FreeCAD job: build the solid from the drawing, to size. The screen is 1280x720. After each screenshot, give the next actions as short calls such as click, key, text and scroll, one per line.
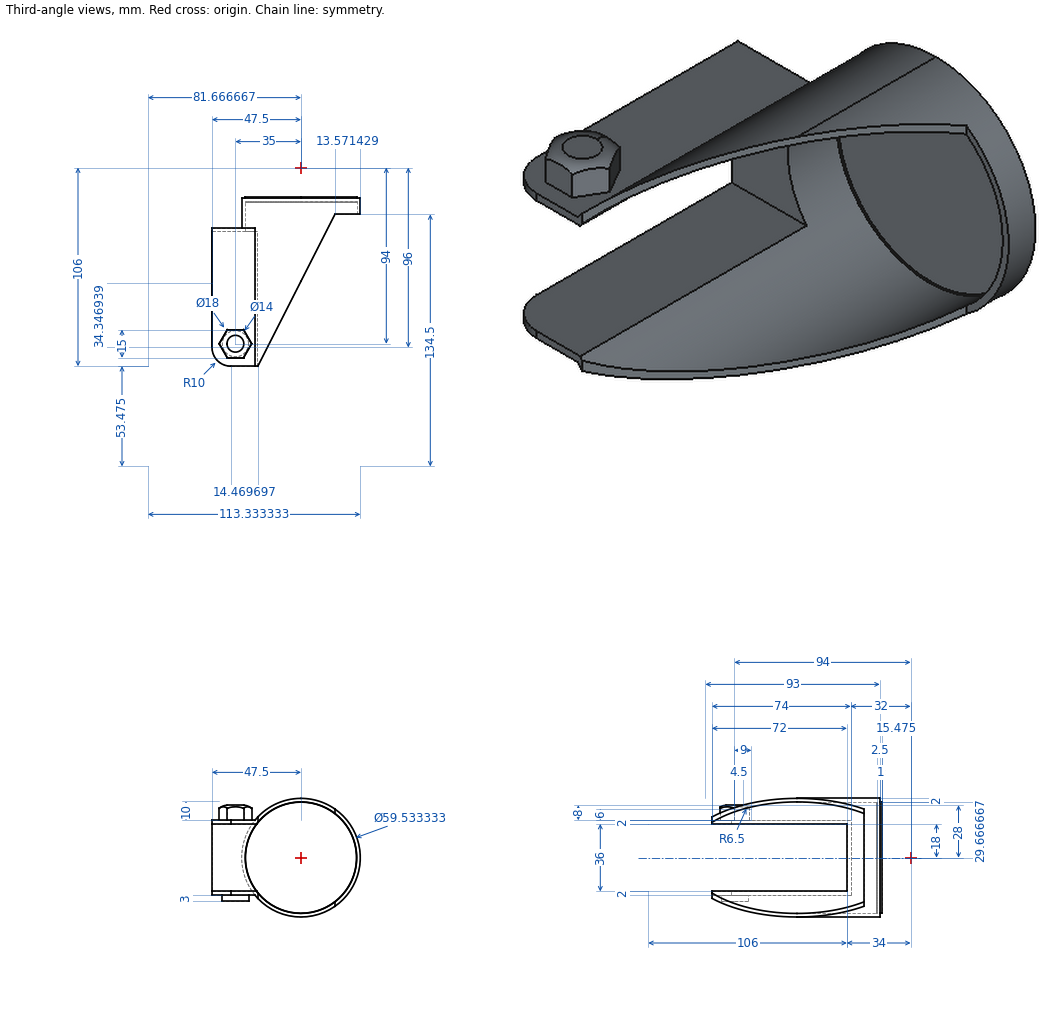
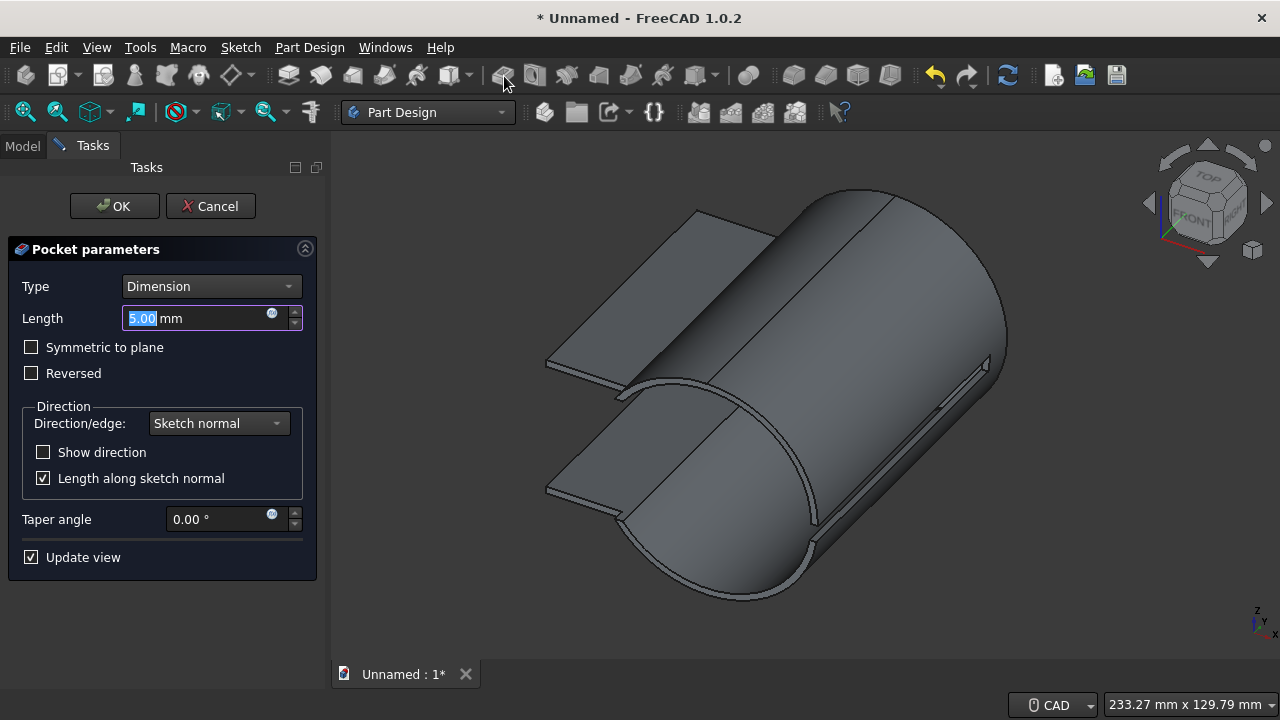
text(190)
key(Tab)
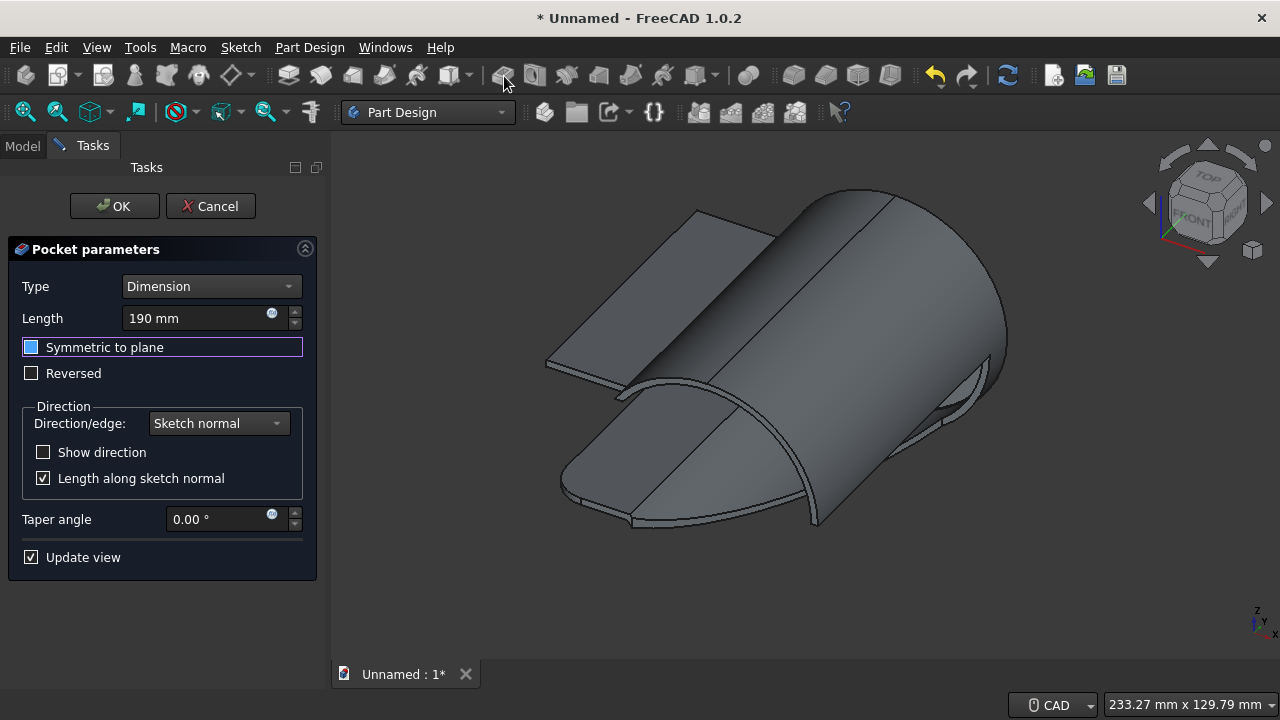
click(30, 347)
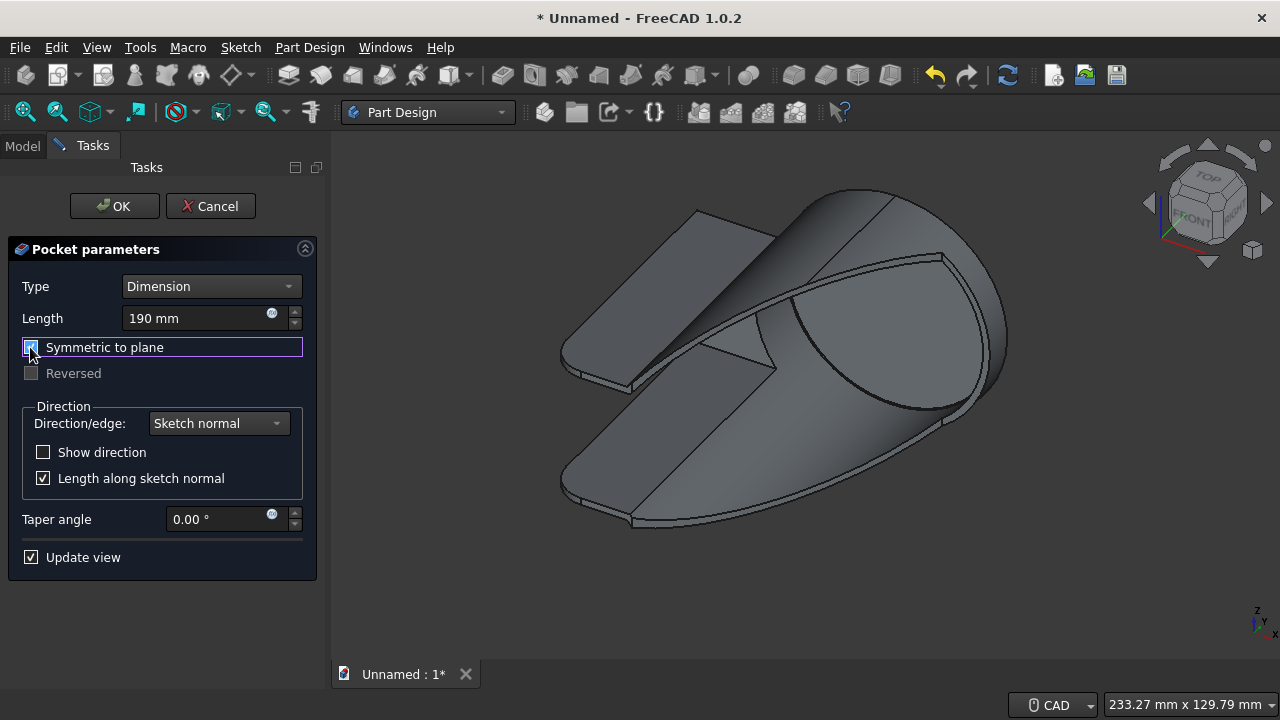
click(115, 206)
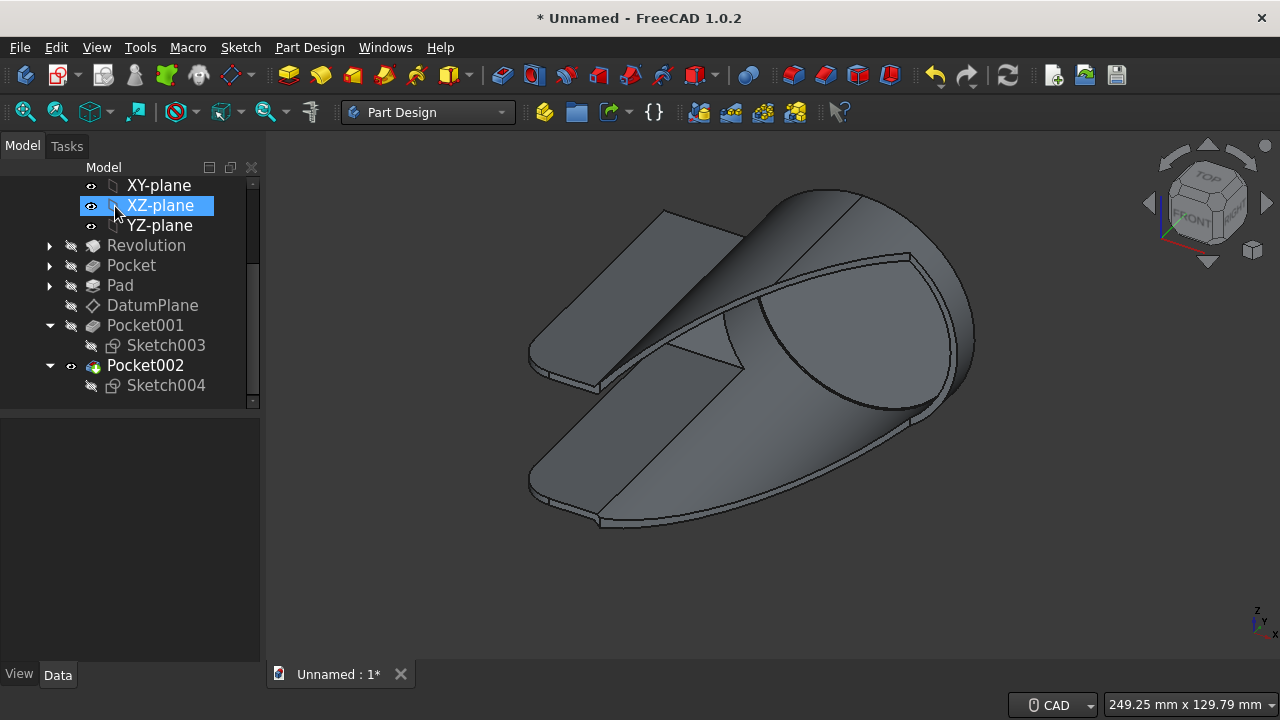
key(5)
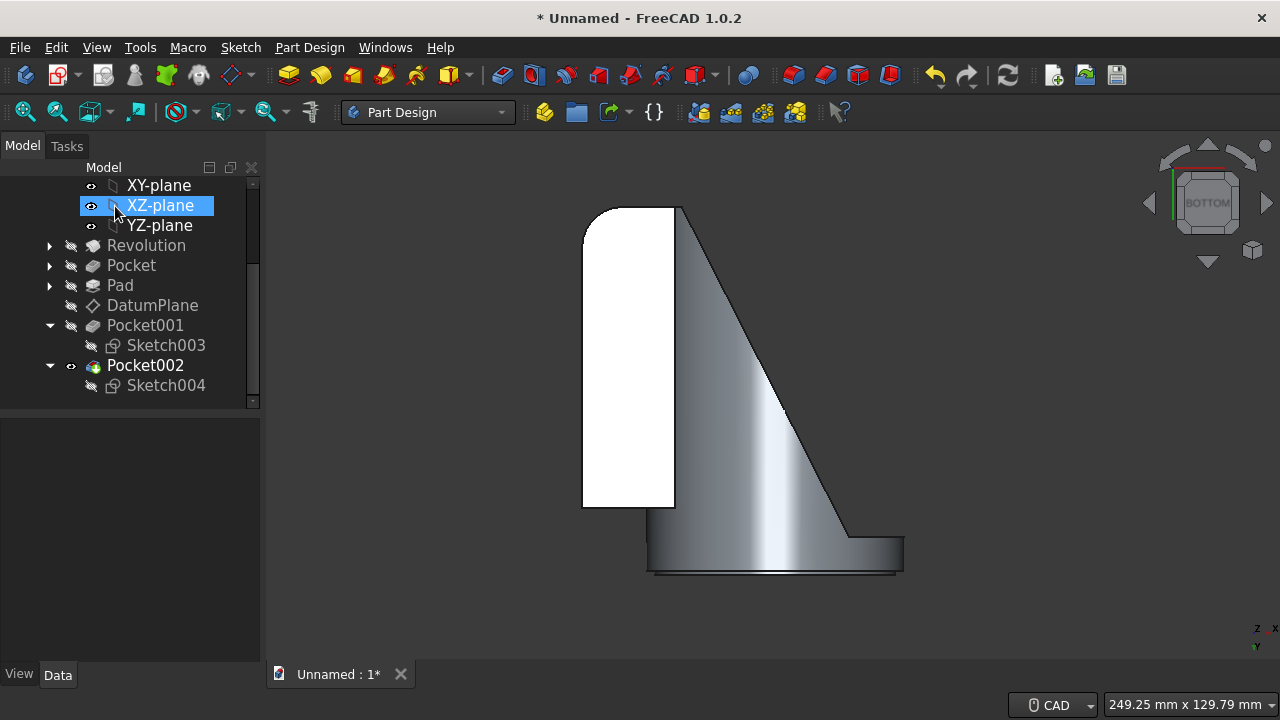
click(629, 443)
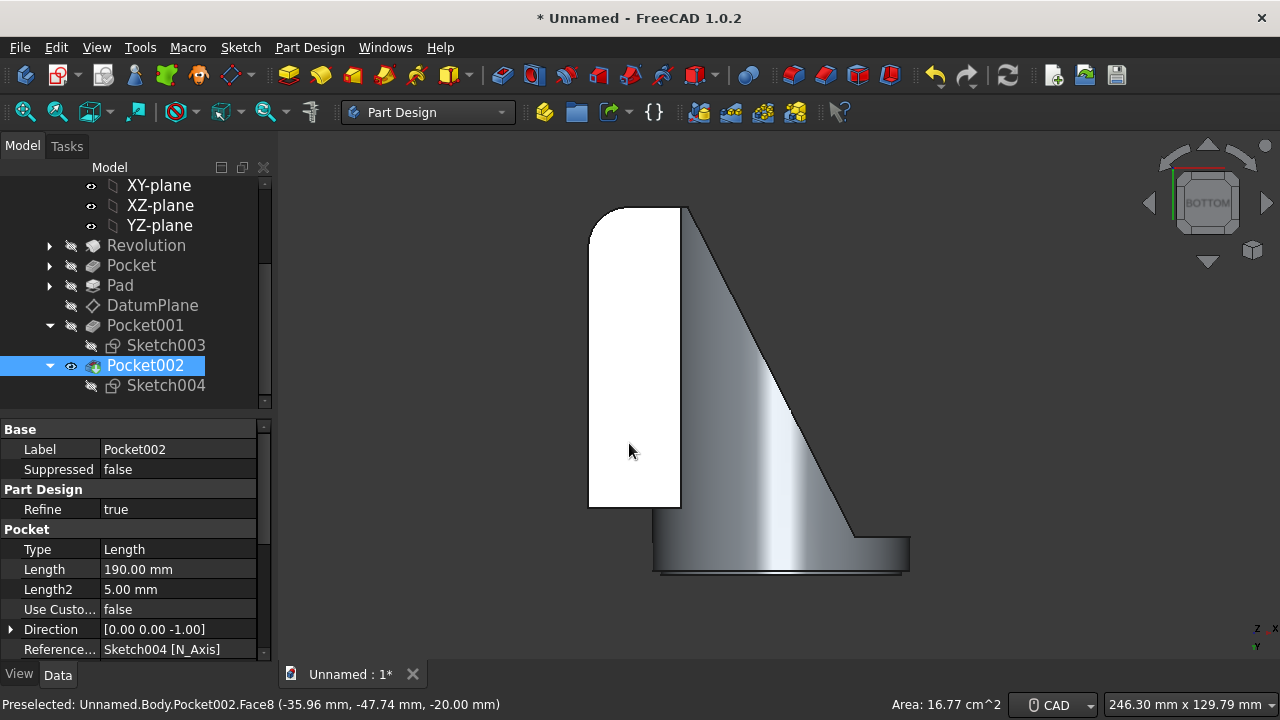
click(58, 76)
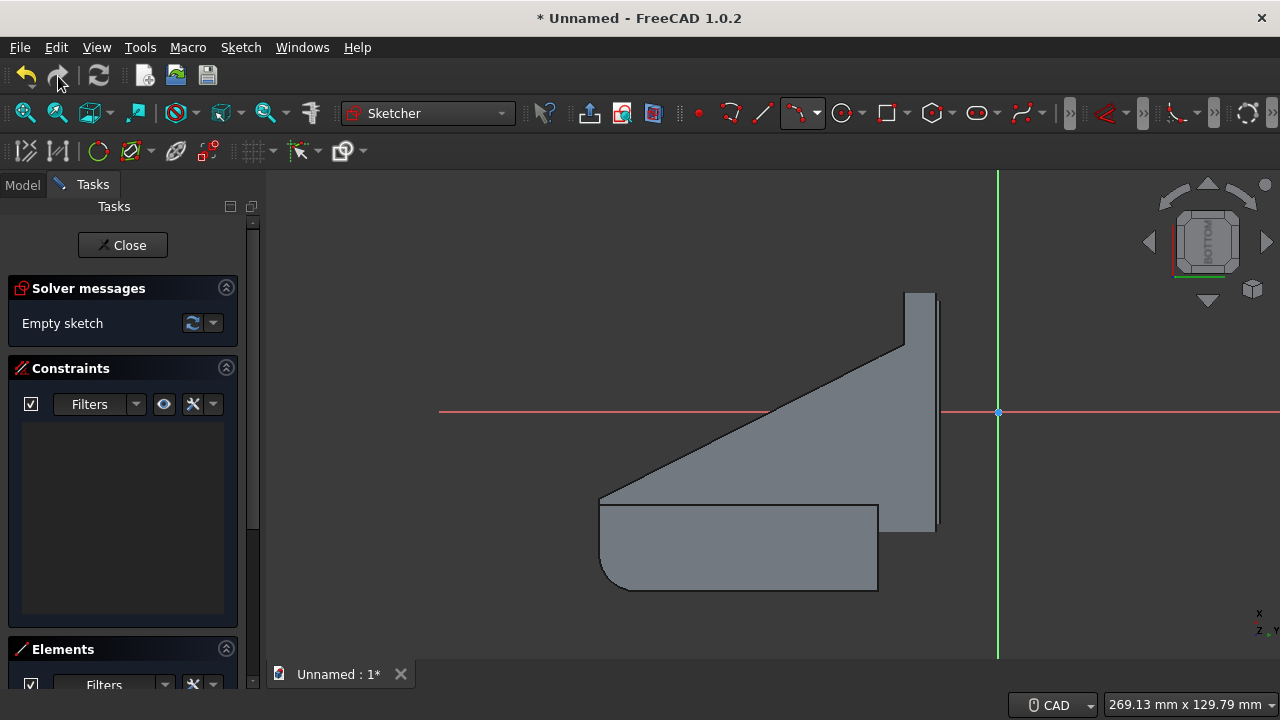
key(q)
key(s)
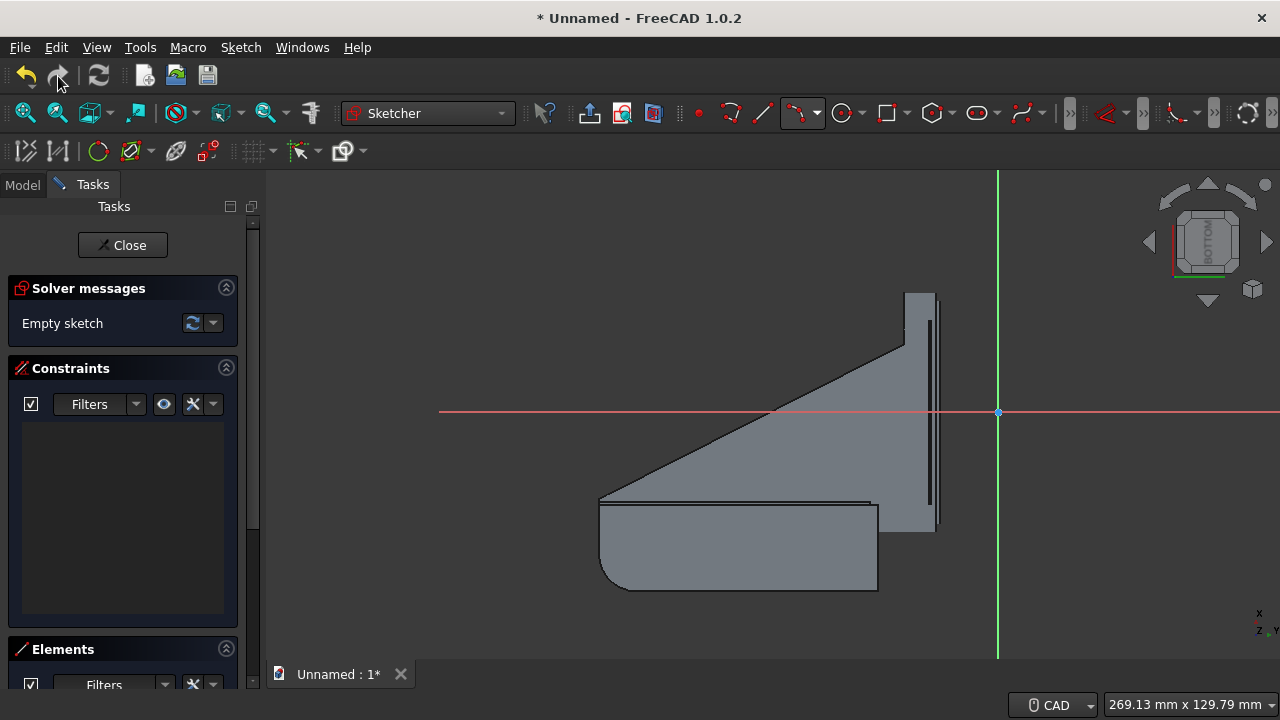
scroll(632, 570, up, 9)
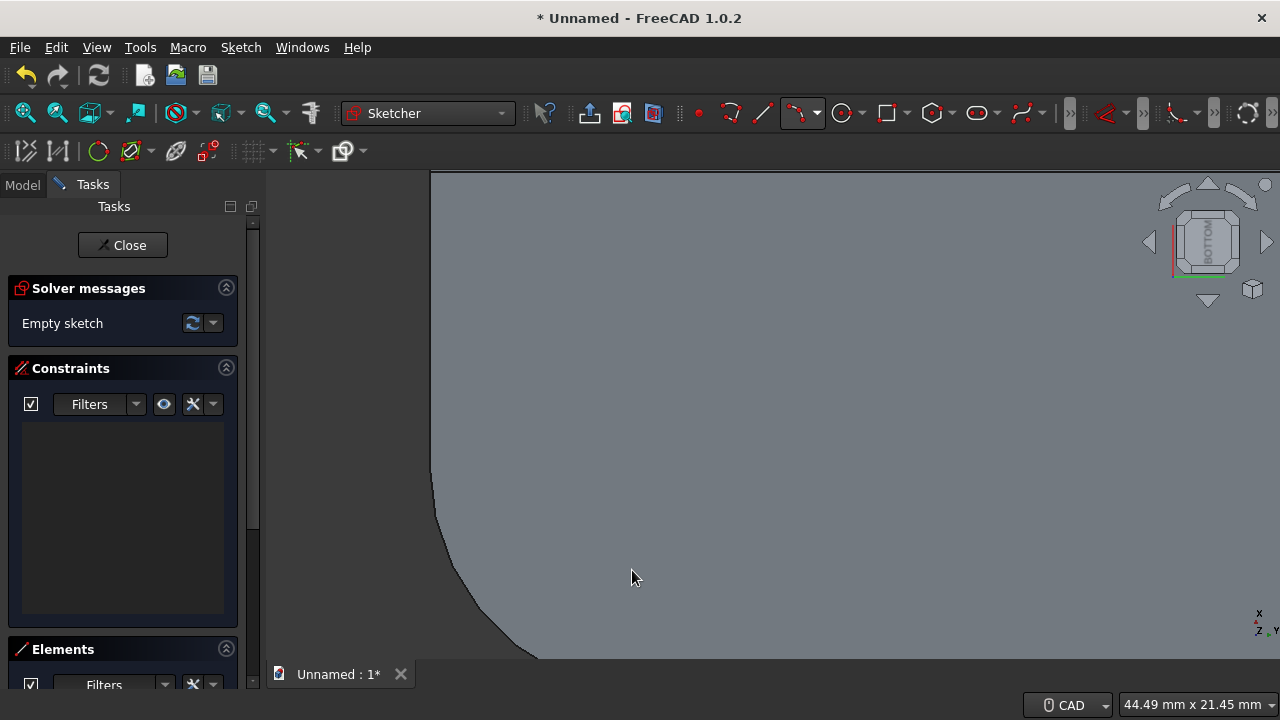
click(842, 114)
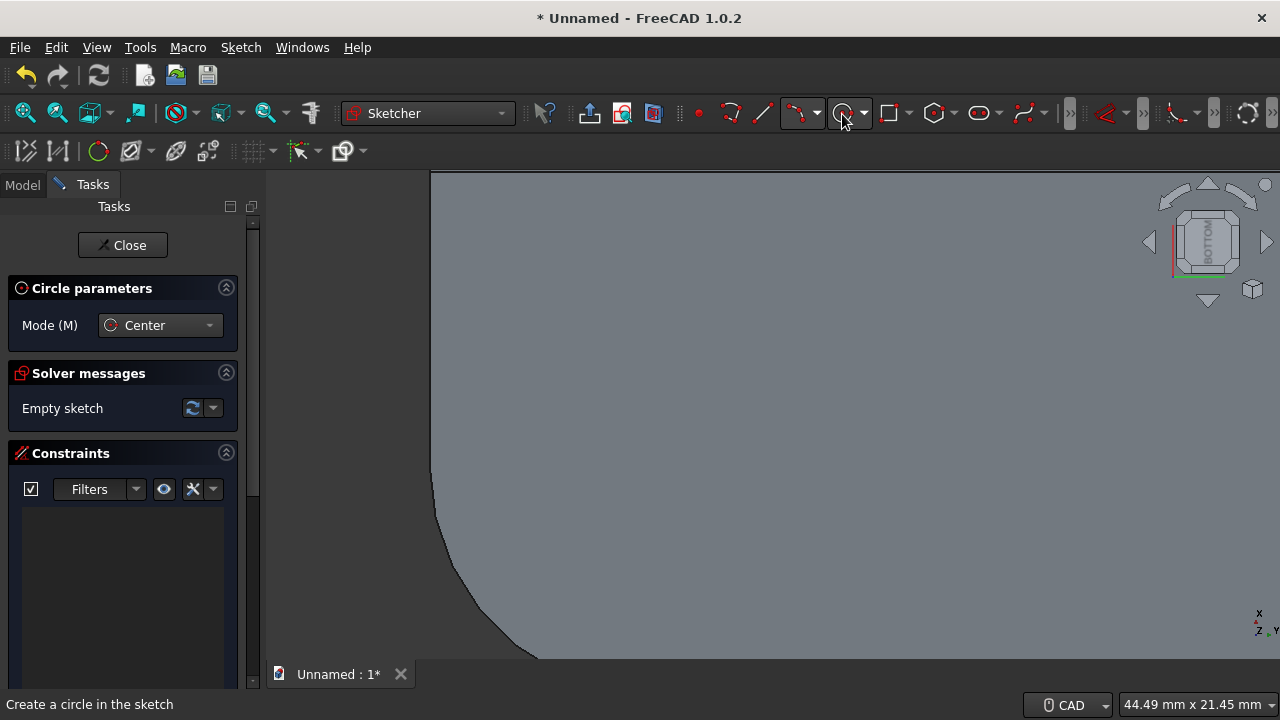
click(703, 410)
click(816, 297)
key(Escape)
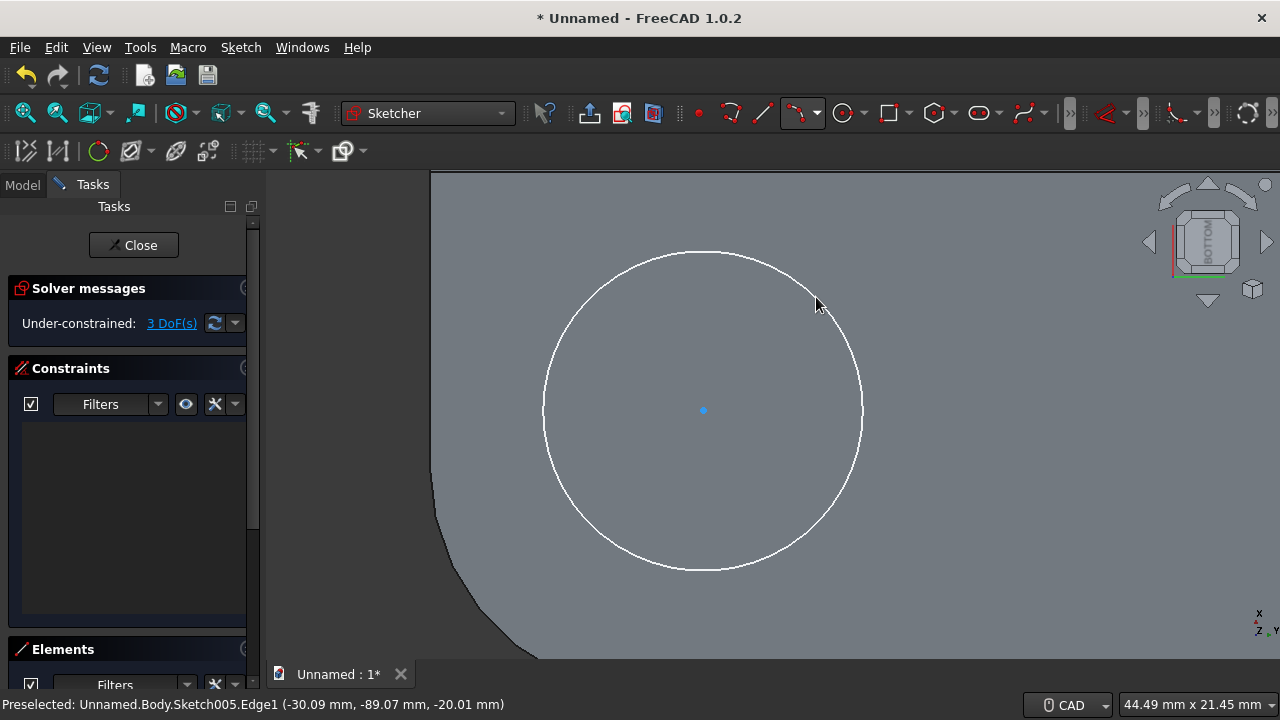
key(d)